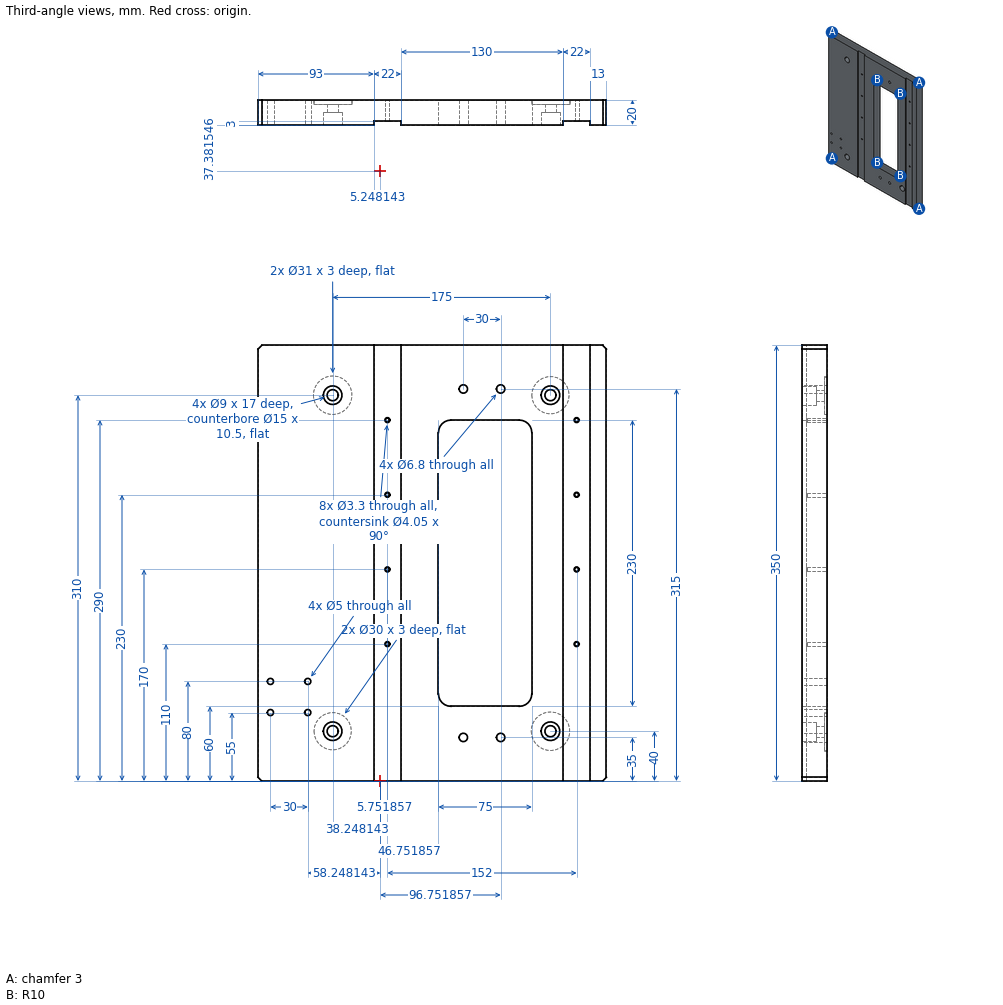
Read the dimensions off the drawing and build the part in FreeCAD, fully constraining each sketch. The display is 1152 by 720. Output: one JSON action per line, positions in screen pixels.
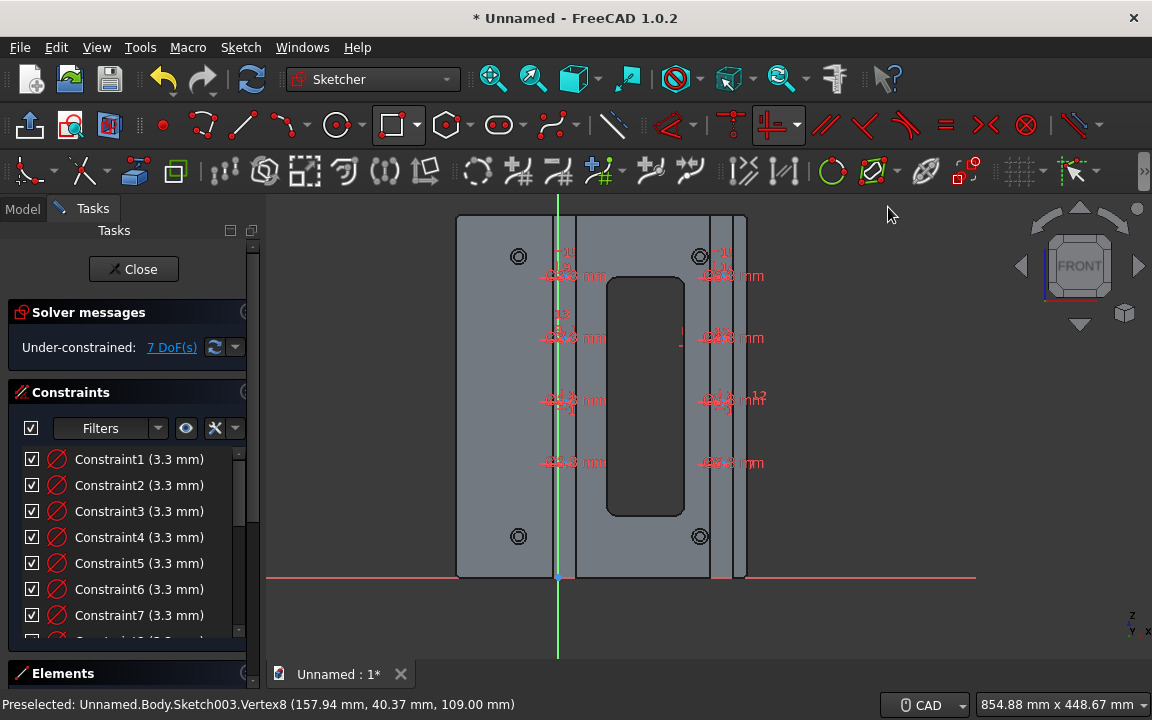
{"action": "left_click", "coordinate": [564, 464]}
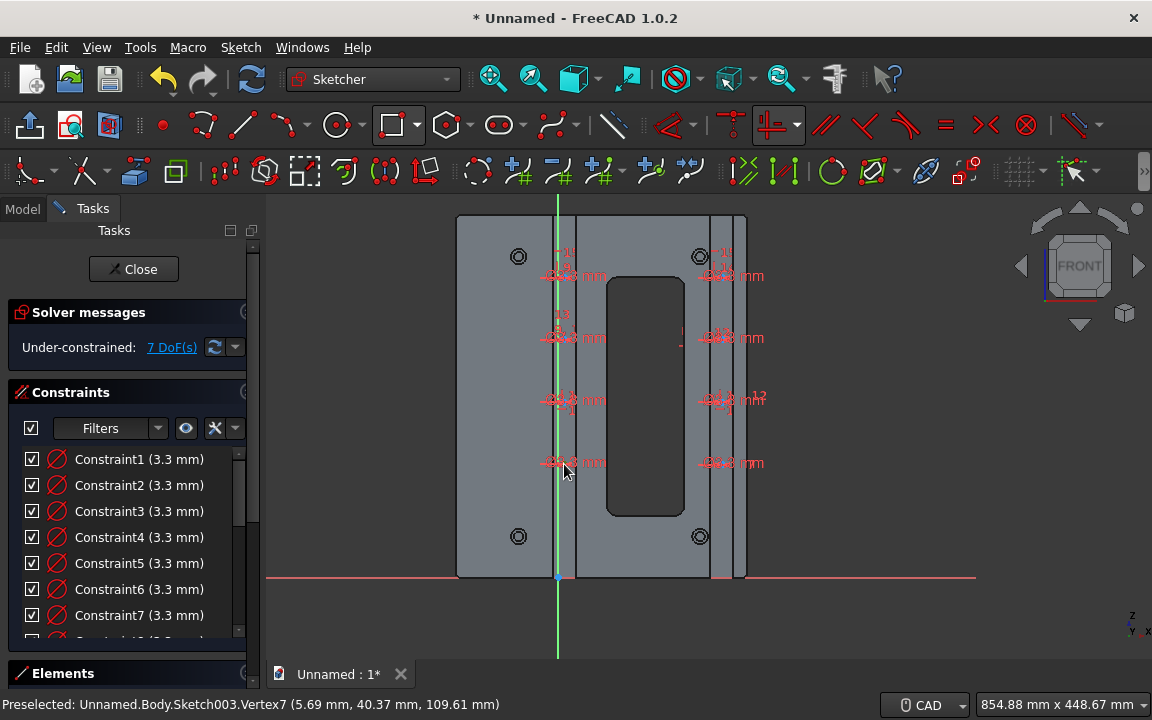
{"action": "left_click", "coordinate": [722, 465]}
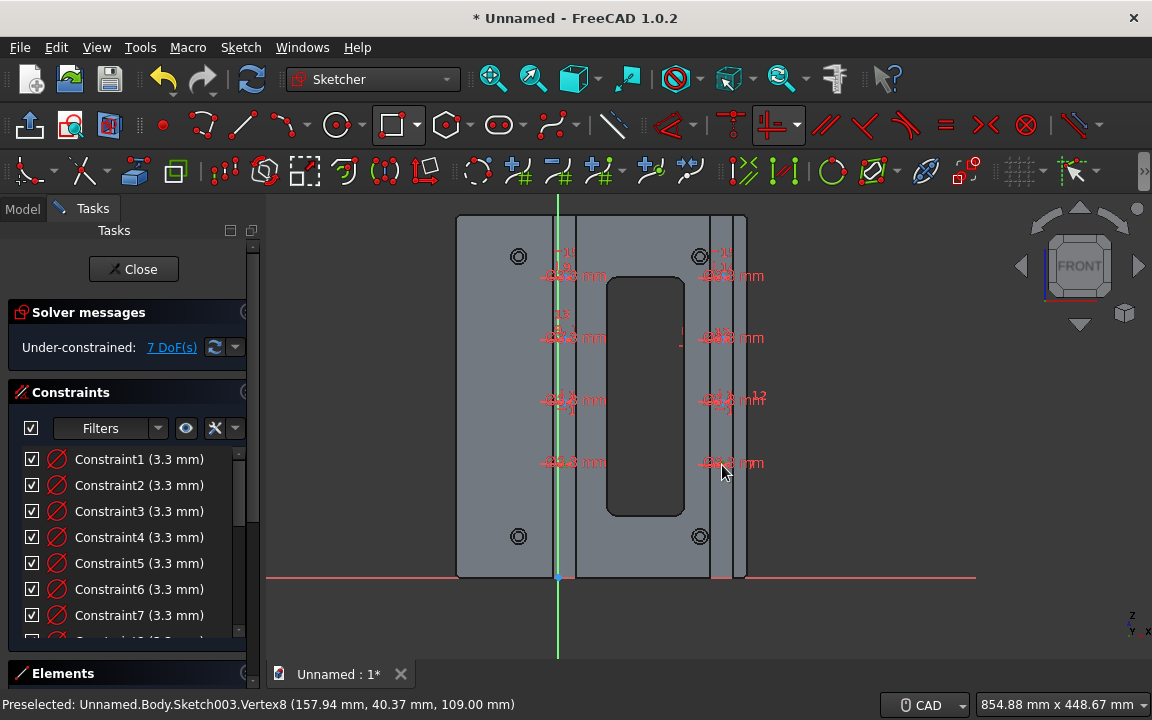
{"action": "key", "text": "h"}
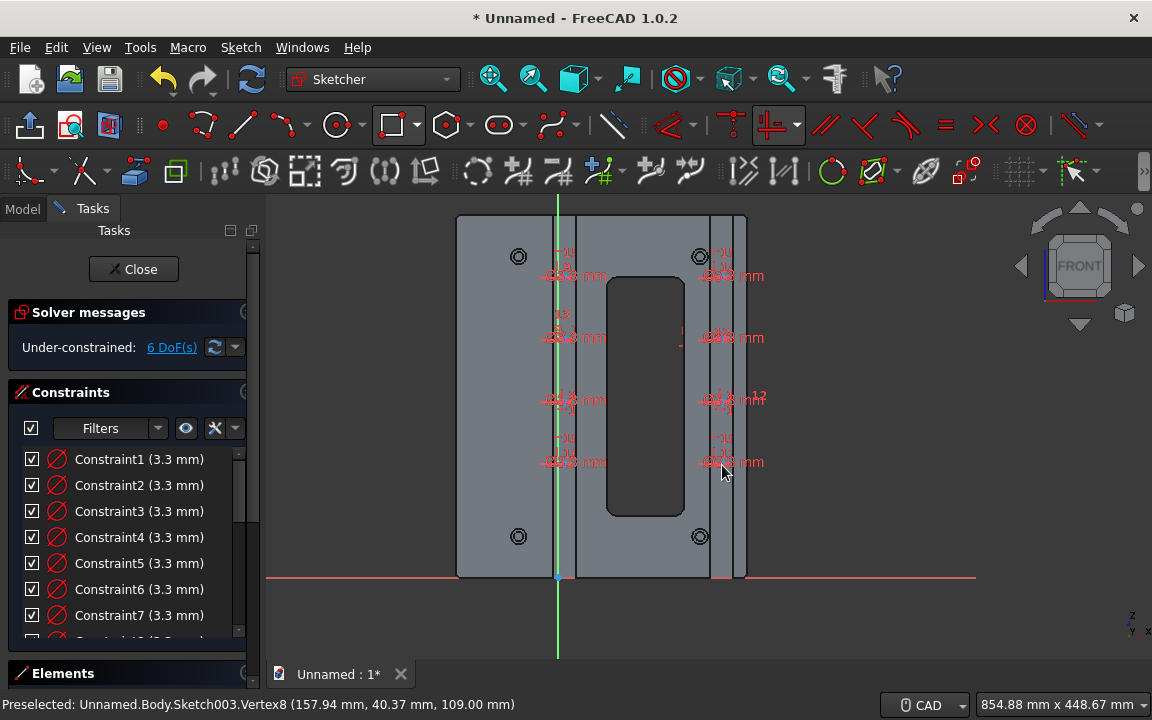
{"action": "left_click", "coordinate": [668, 126]}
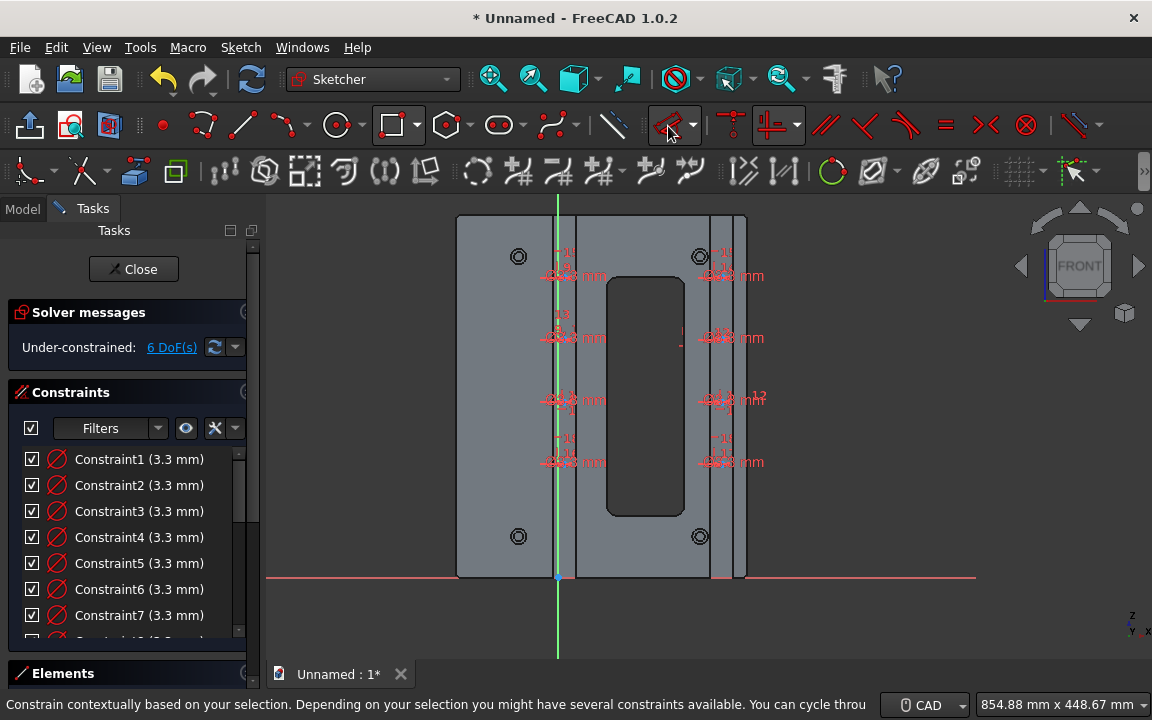
{"action": "left_click", "coordinate": [564, 278]}
{"action": "left_click", "coordinate": [524, 428]}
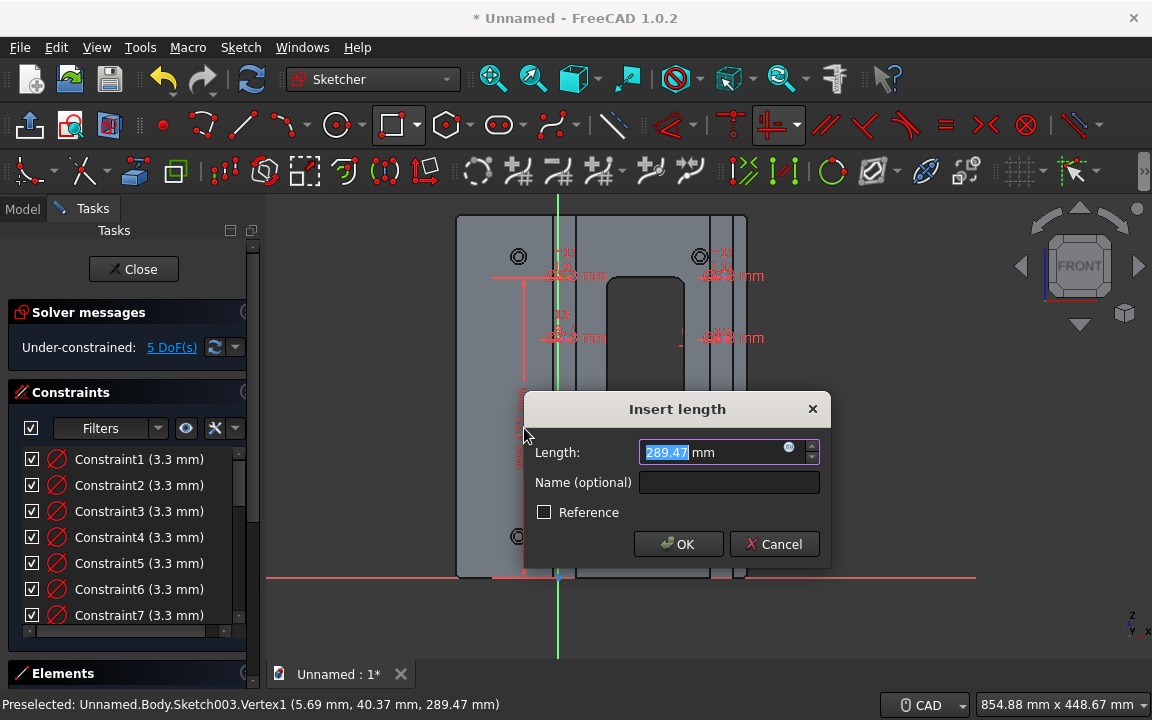
{"action": "type", "text": "290"}
{"action": "key", "text": "Return"}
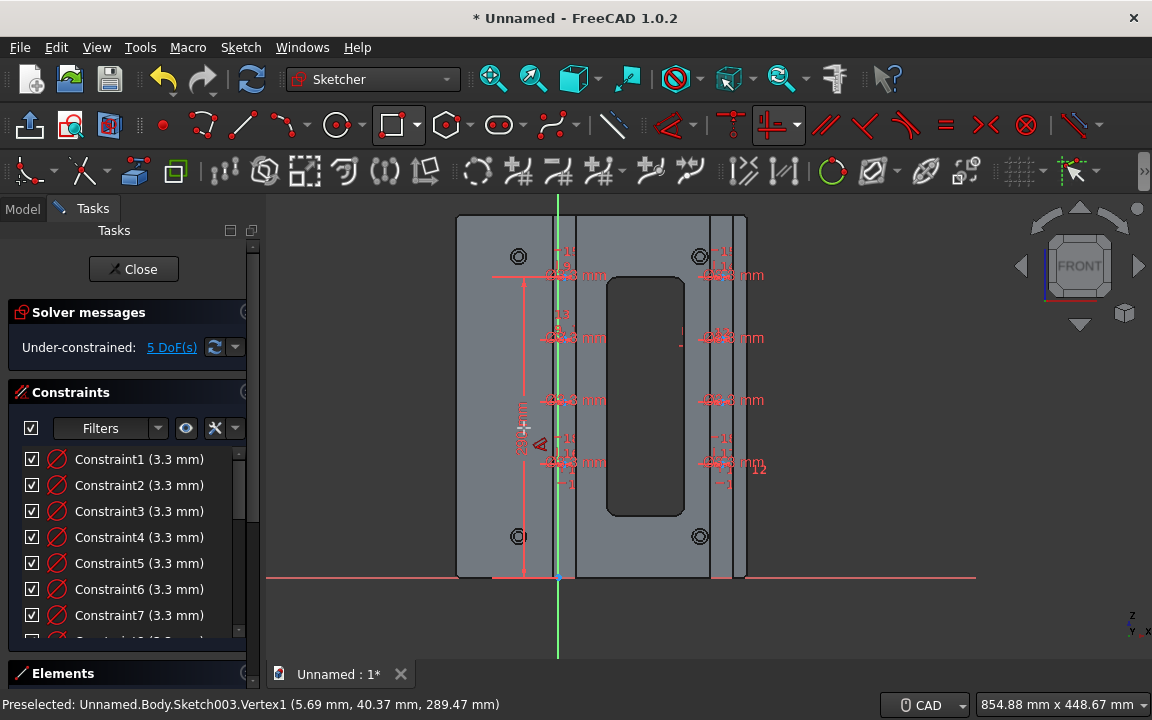
{"action": "left_click", "coordinate": [564, 340]}
{"action": "left_click", "coordinate": [524, 459]}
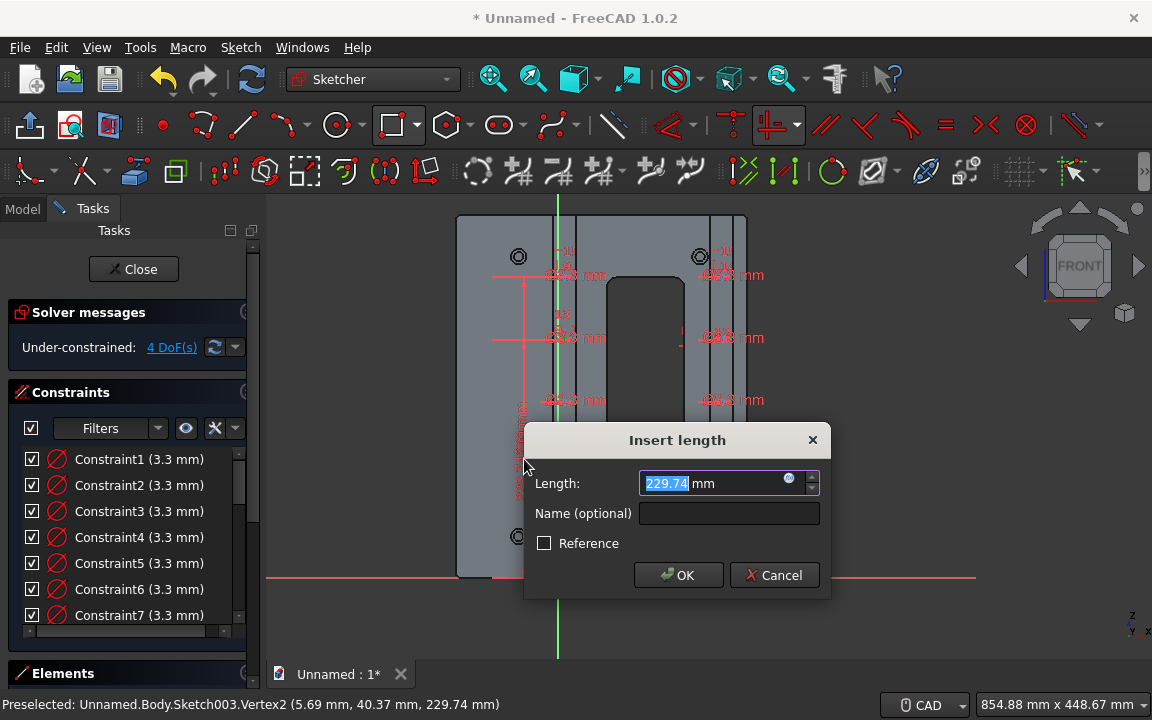
{"action": "type", "text": "230"}
{"action": "key", "text": "Return"}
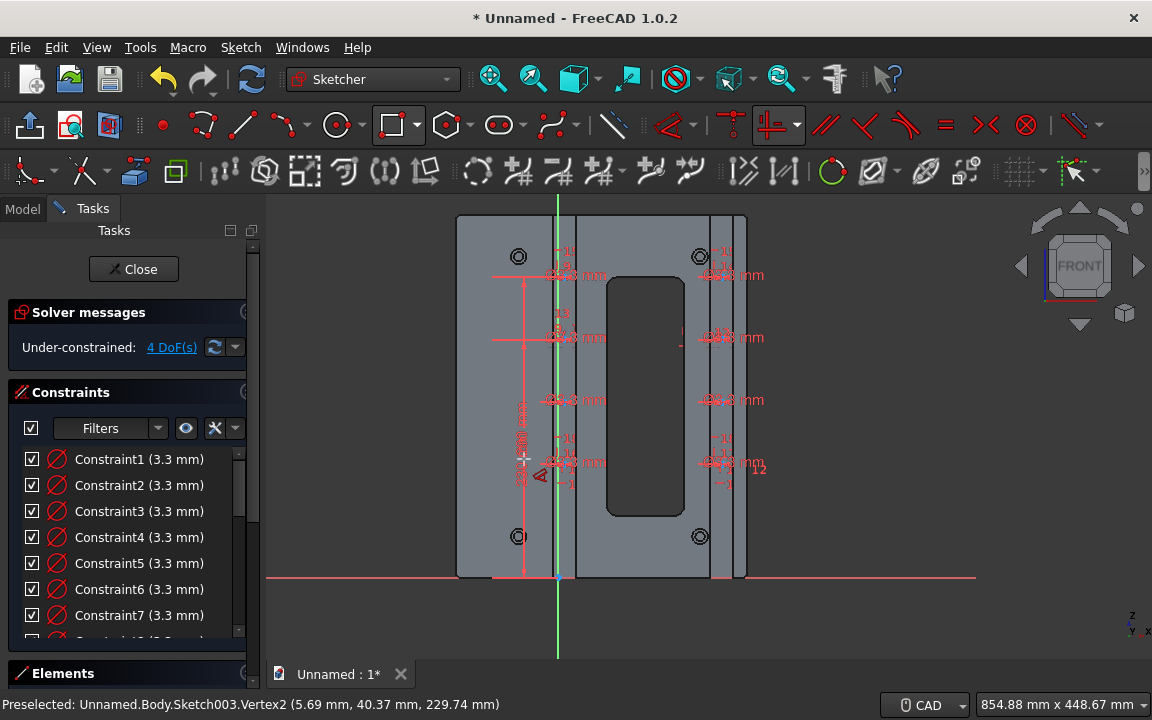
{"action": "left_click", "coordinate": [564, 402]}
{"action": "left_click", "coordinate": [524, 490]}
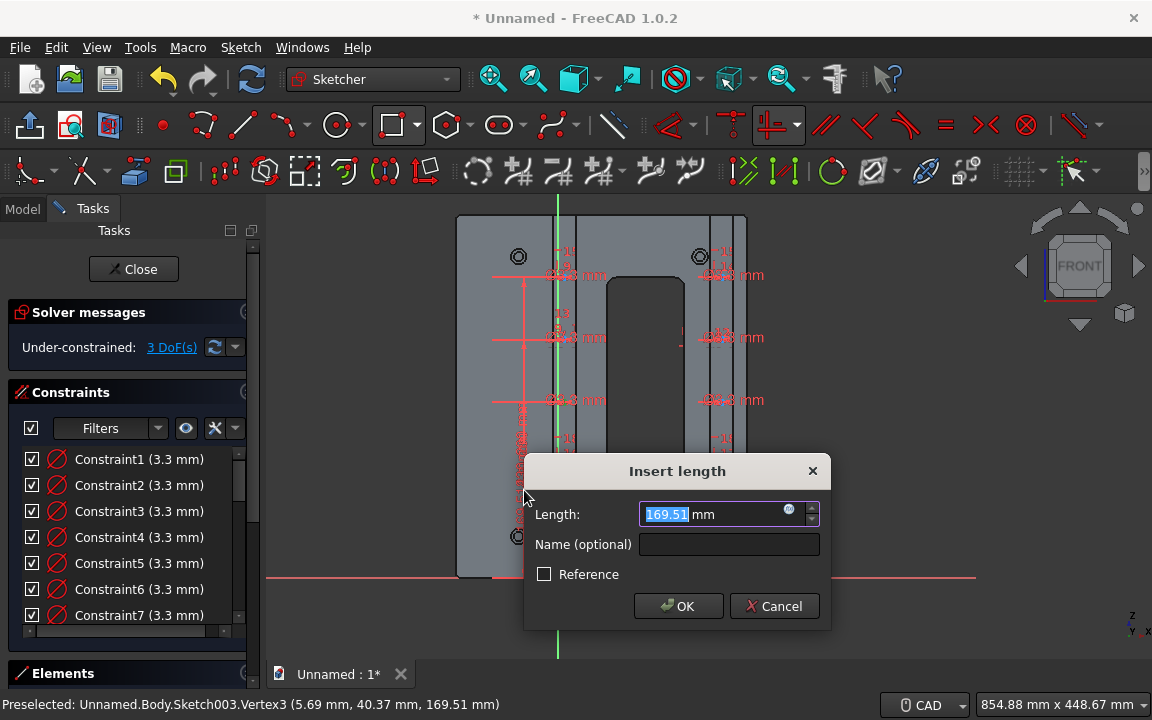
{"action": "type", "text": "170"}
{"action": "key", "text": "Return"}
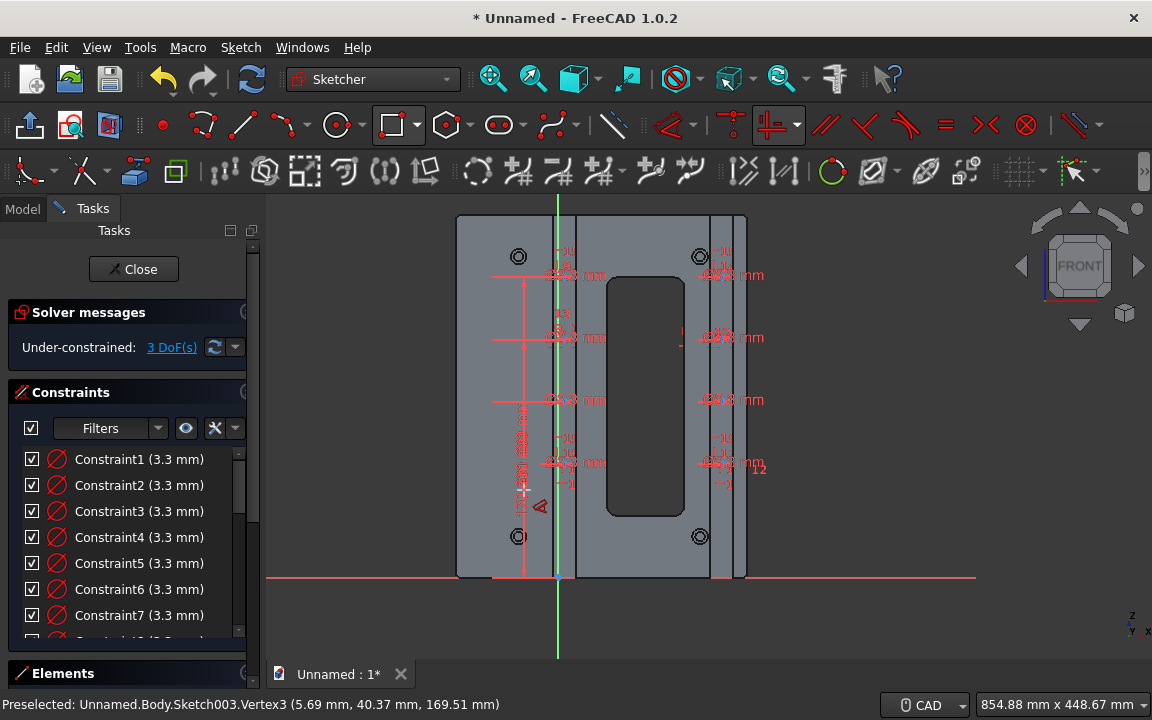
{"action": "left_click", "coordinate": [564, 464]}
{"action": "left_click", "coordinate": [524, 521]}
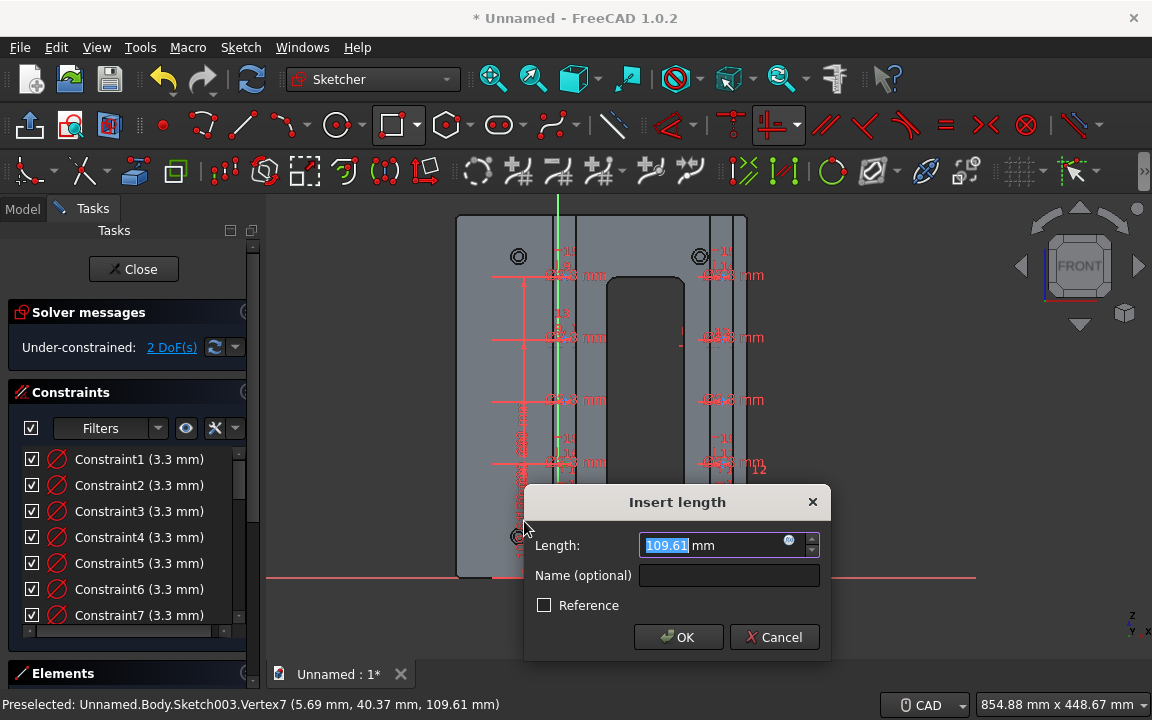
{"action": "type", "text": "110"}
{"action": "key", "text": "Return"}